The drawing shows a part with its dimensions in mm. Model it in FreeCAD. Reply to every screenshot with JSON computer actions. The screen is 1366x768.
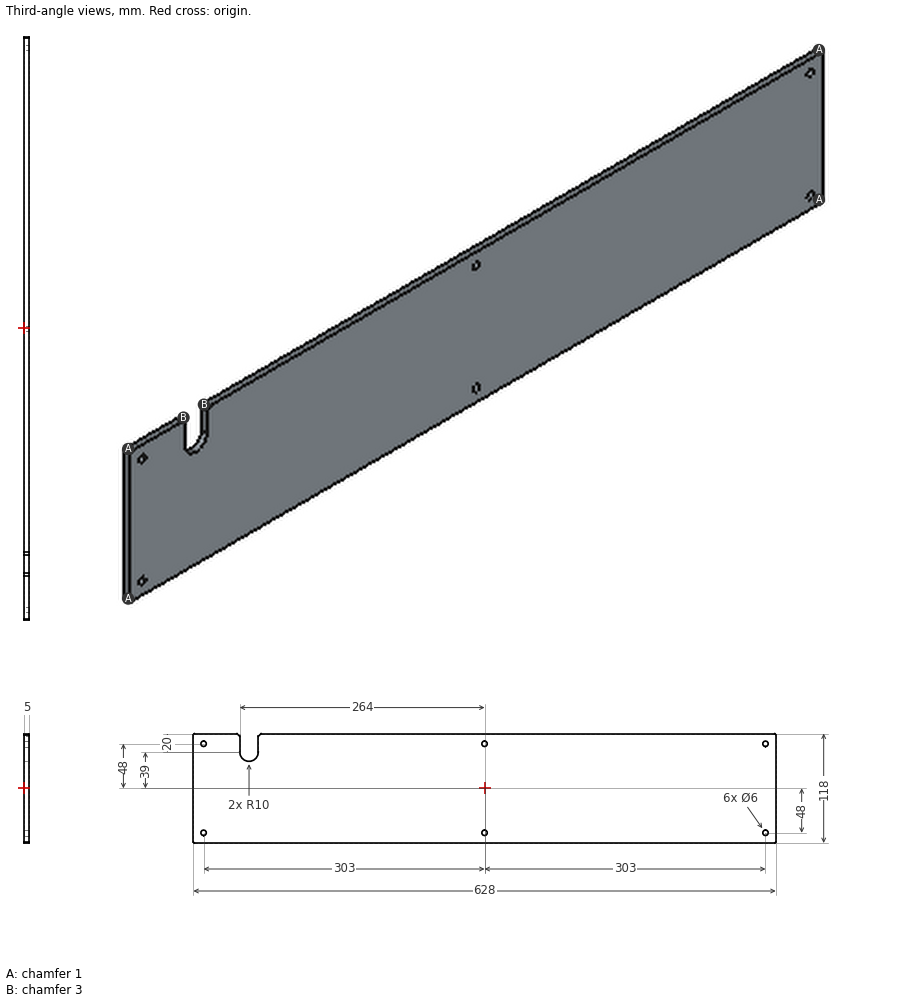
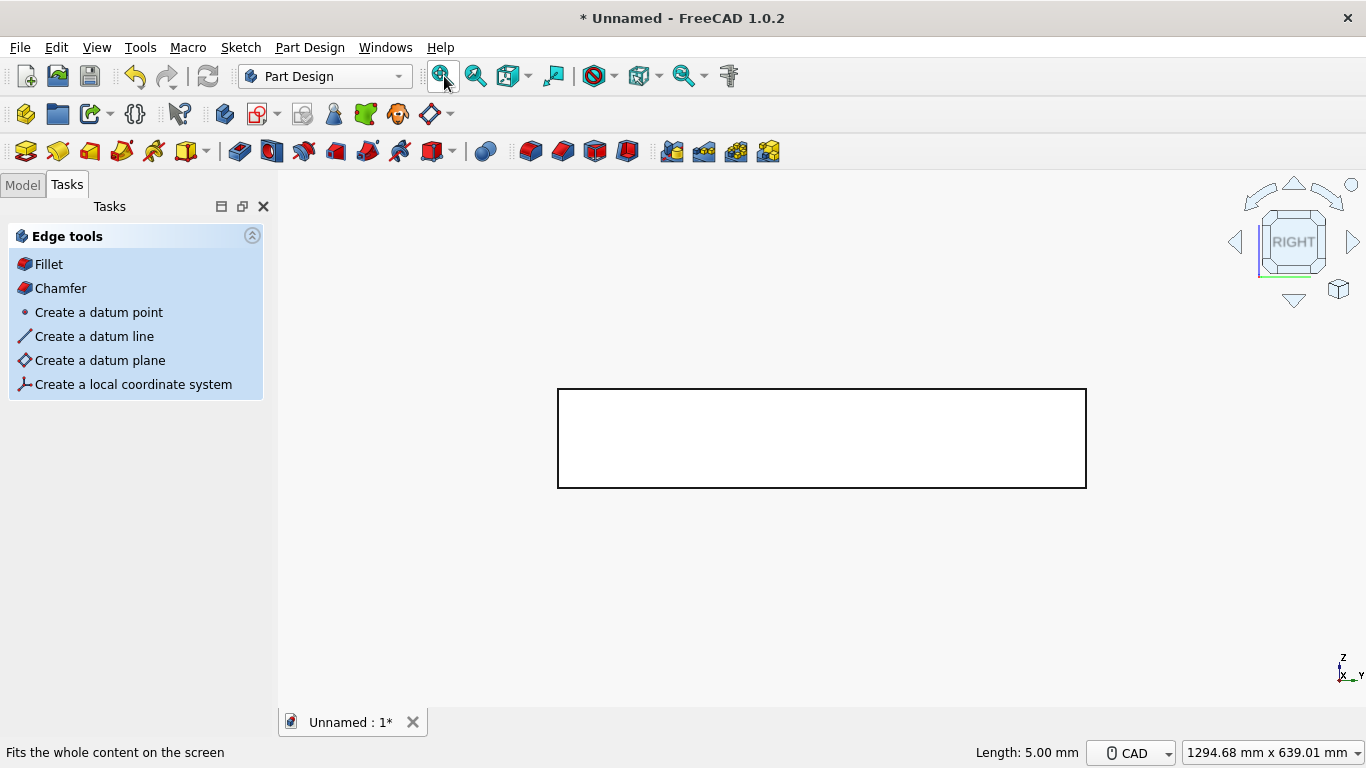
{"action": "key", "text": "5"}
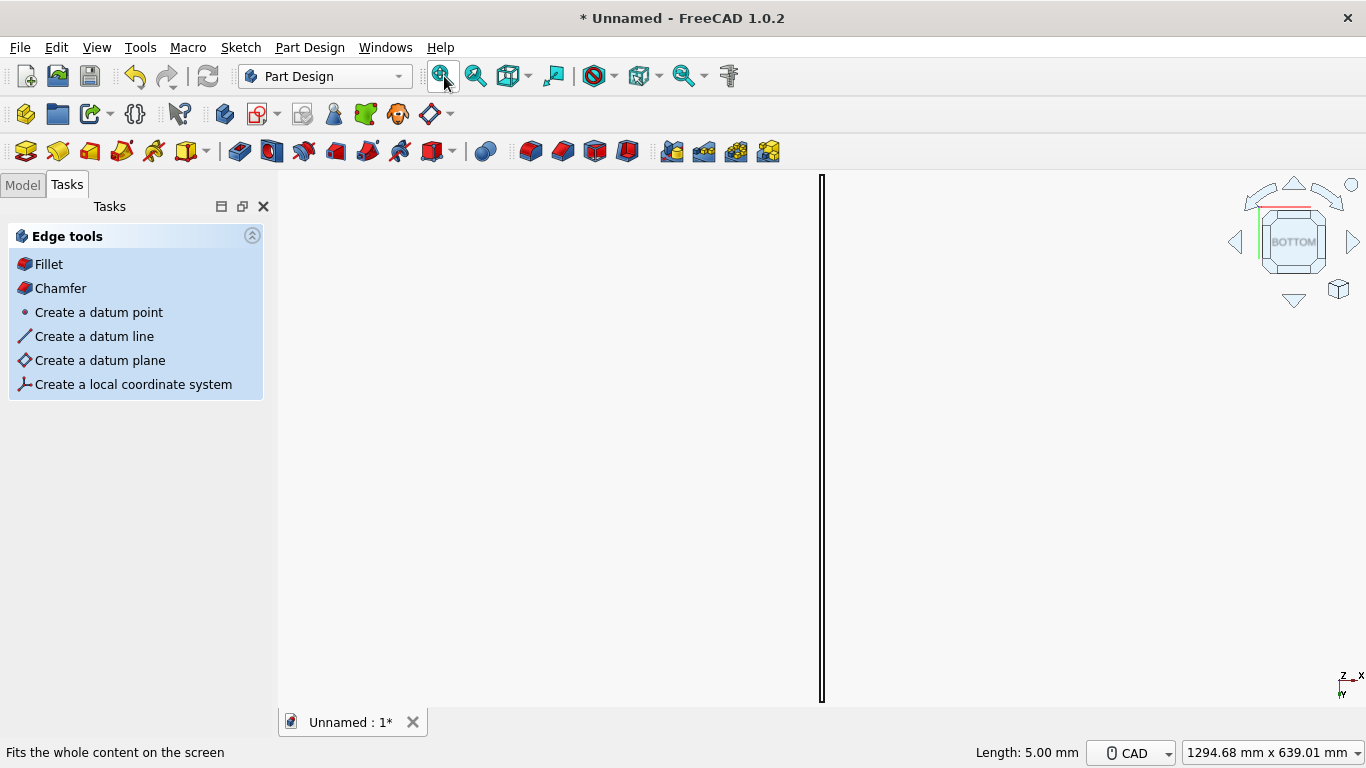
{"action": "key", "text": "4"}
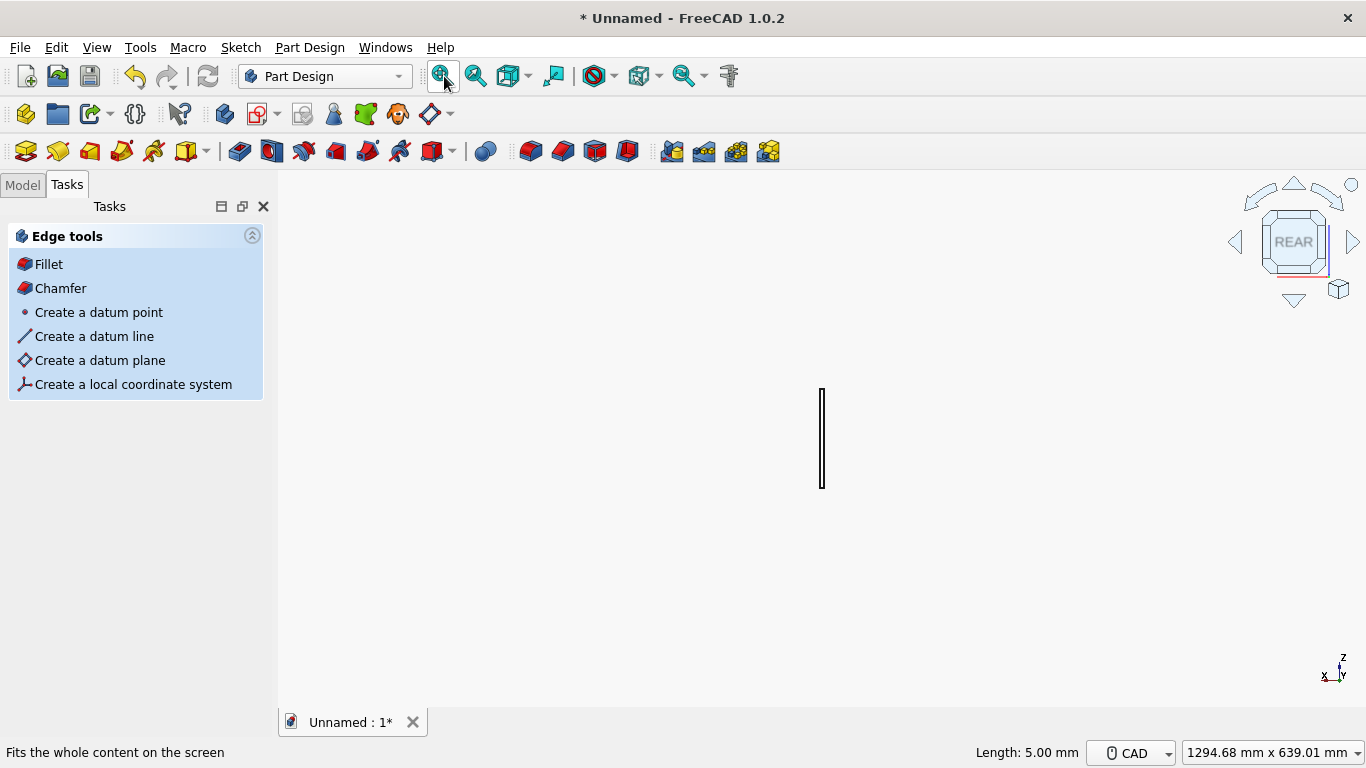
{"action": "left_click", "coordinate": [444, 76]}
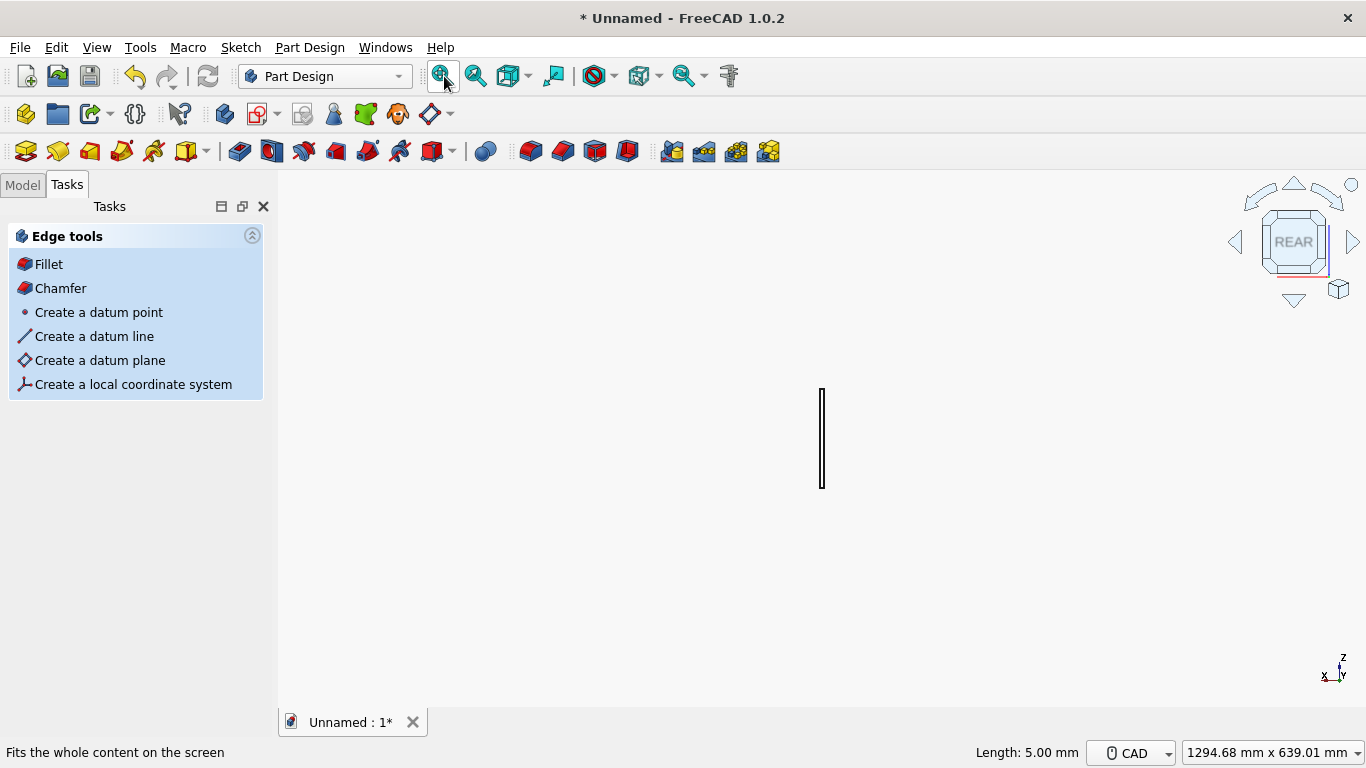
{"action": "scroll", "coordinate": [822, 388], "scroll_direction": "up", "scroll_amount": 12}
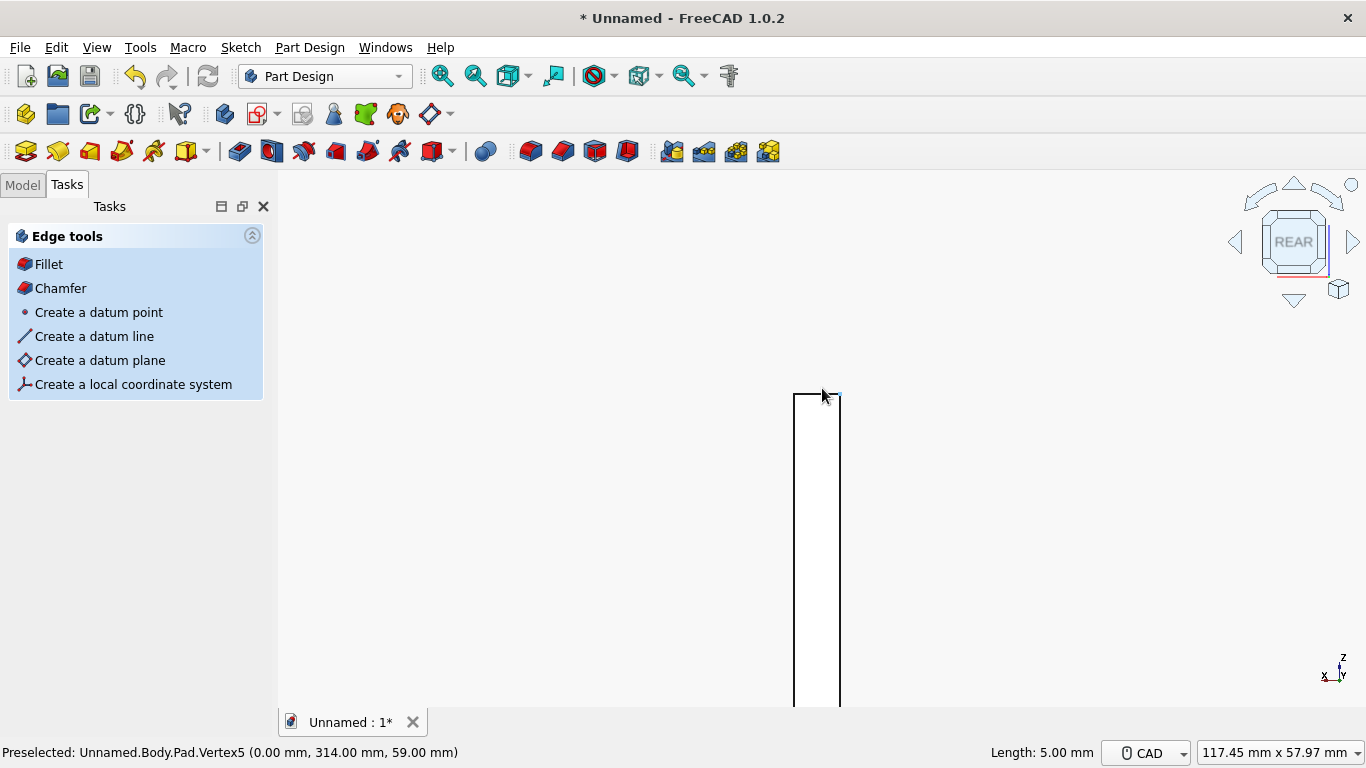
{"action": "left_click", "coordinate": [817, 393], "text": "ctrl"}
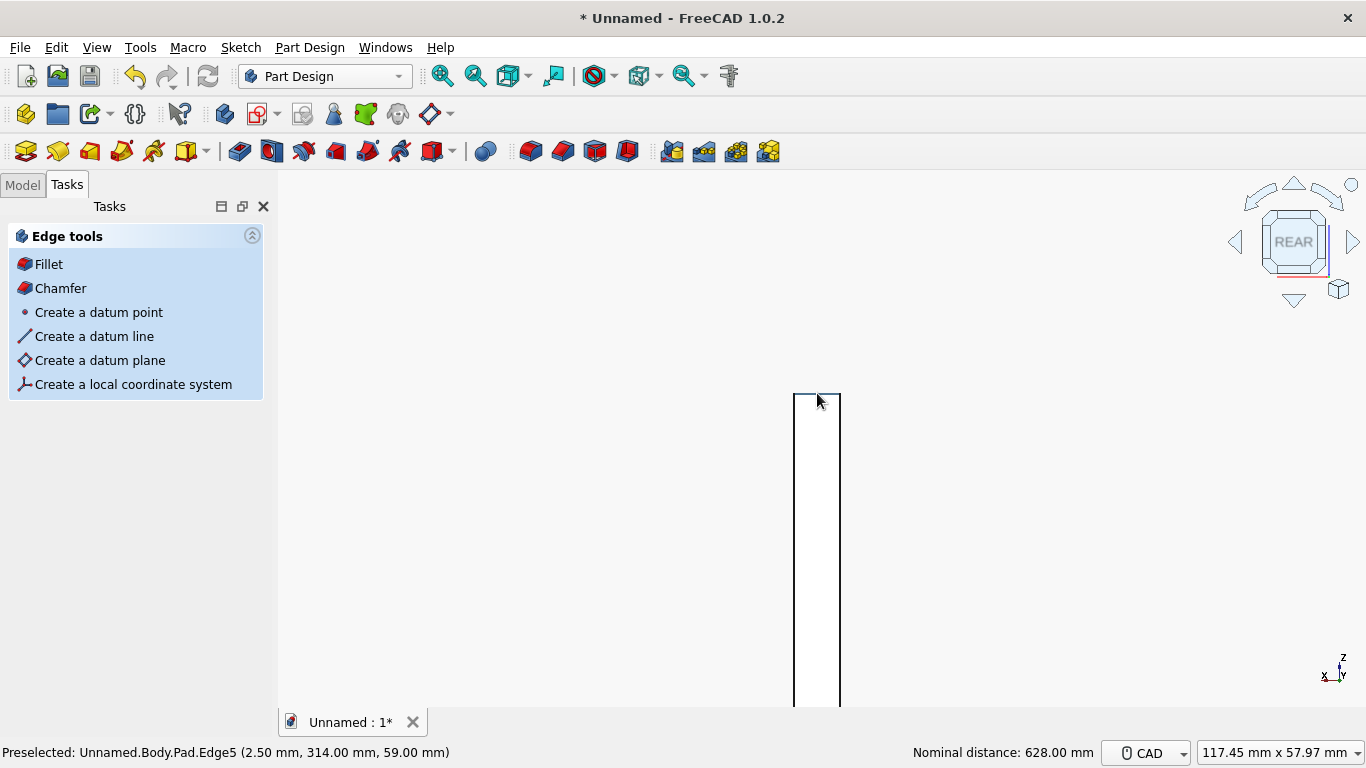
{"action": "left_click", "coordinate": [444, 76]}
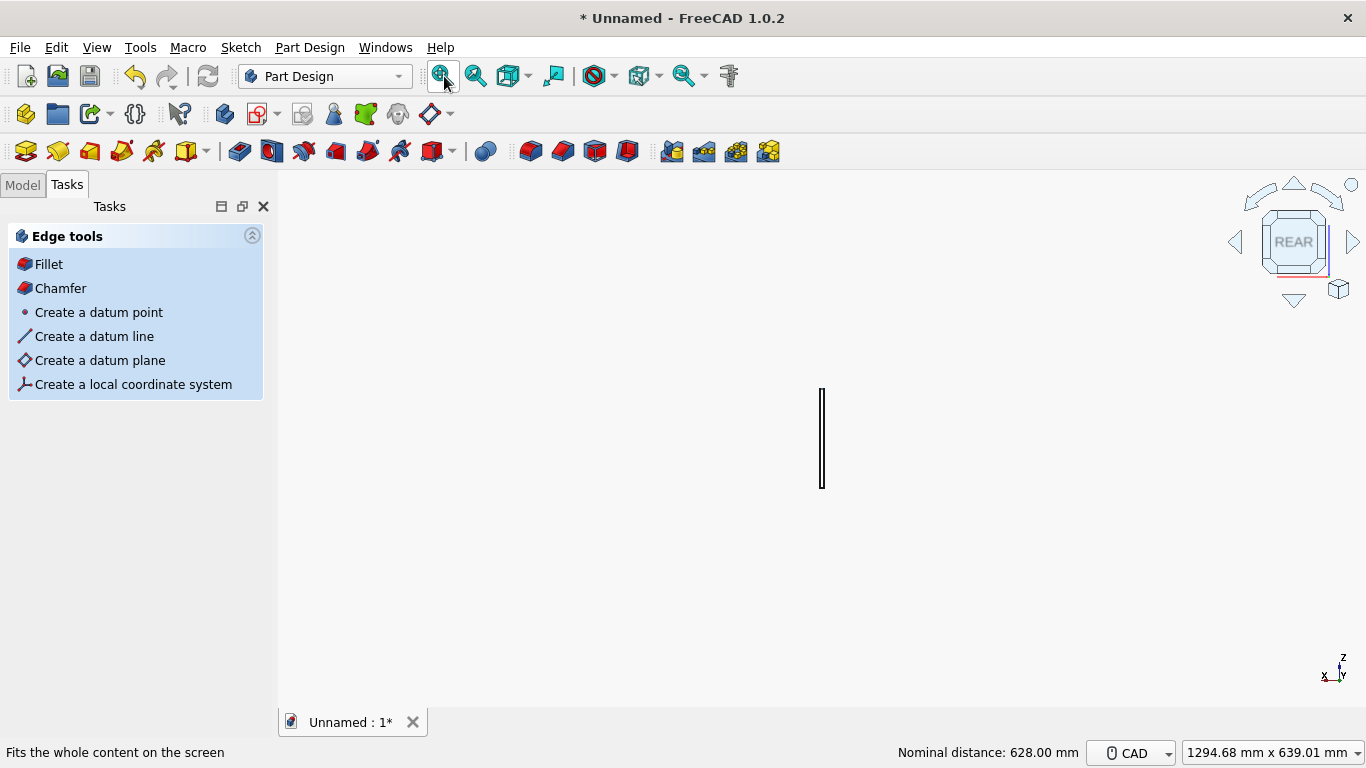
{"action": "key", "text": "6"}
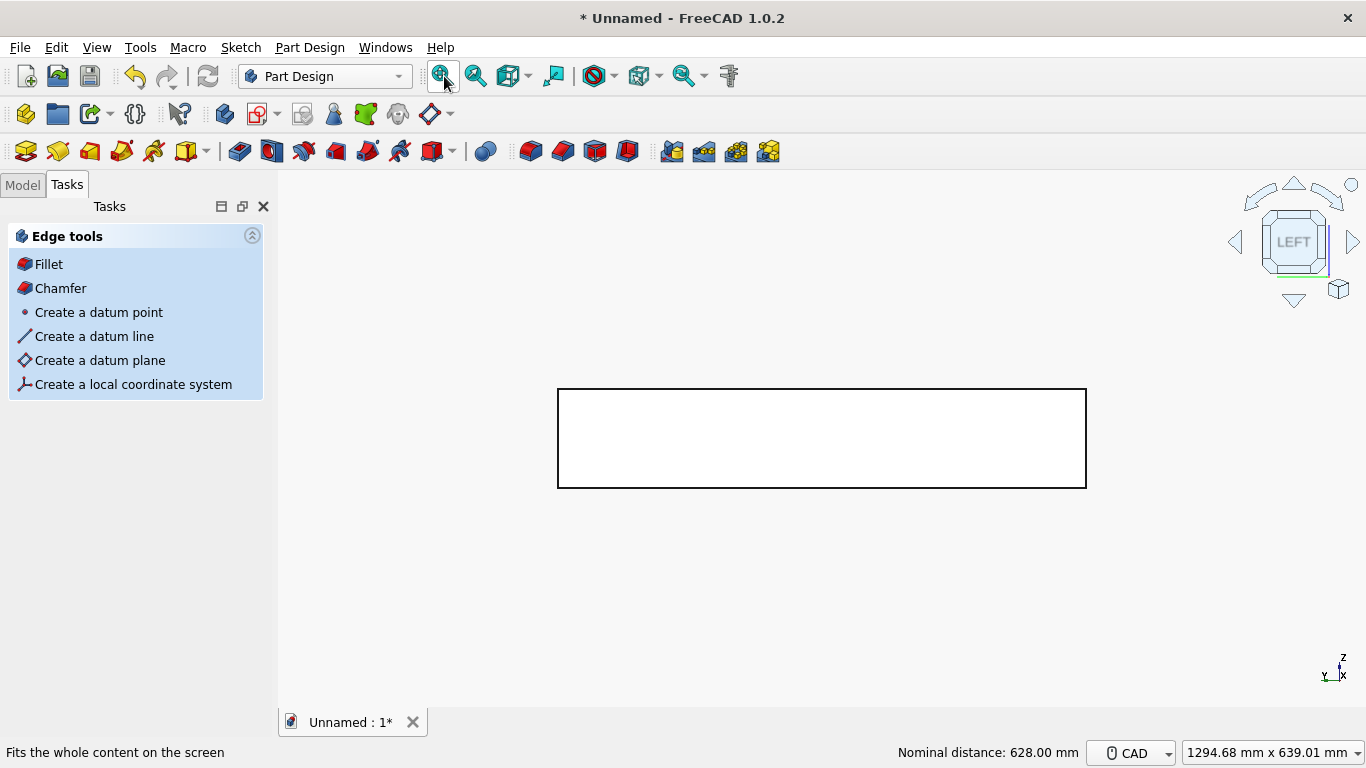
{"action": "scroll", "coordinate": [558, 487], "scroll_direction": "up", "scroll_amount": 12}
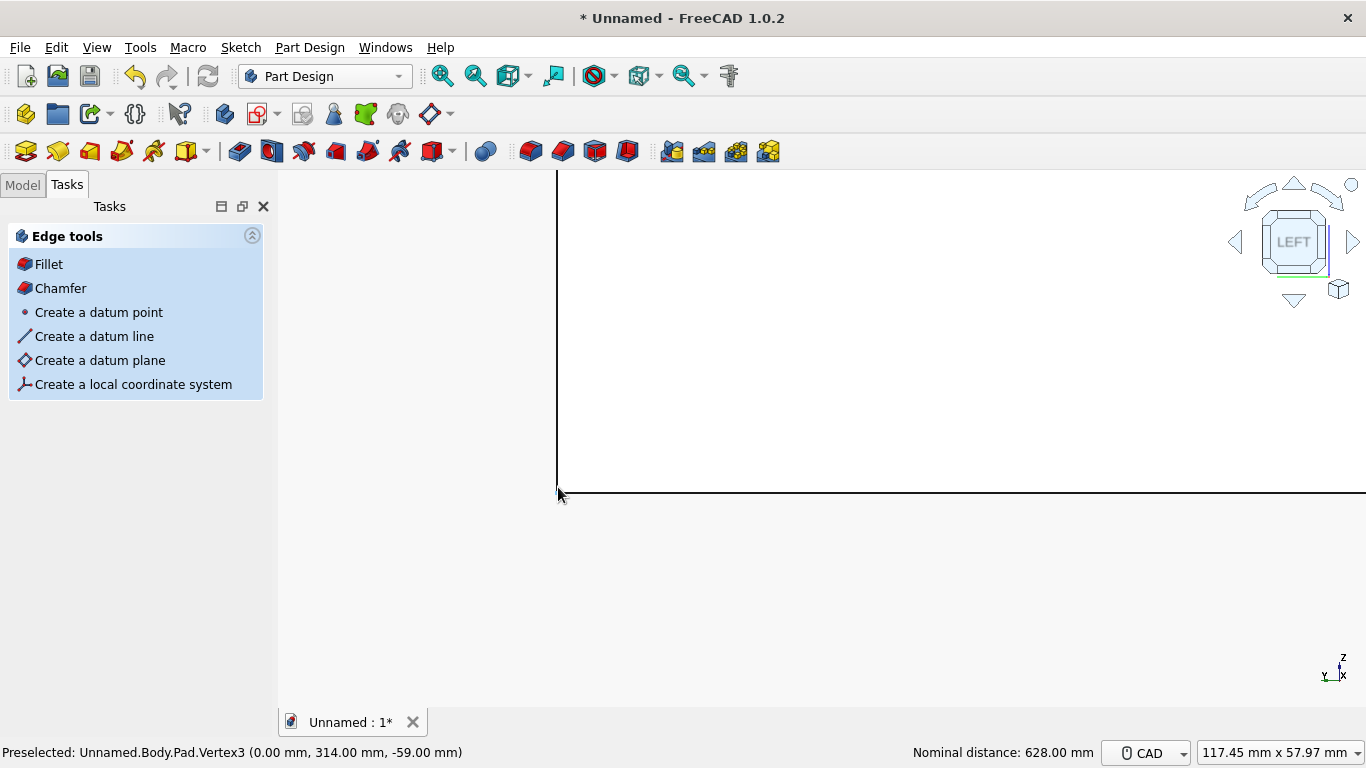
{"action": "left_click", "coordinate": [444, 76]}